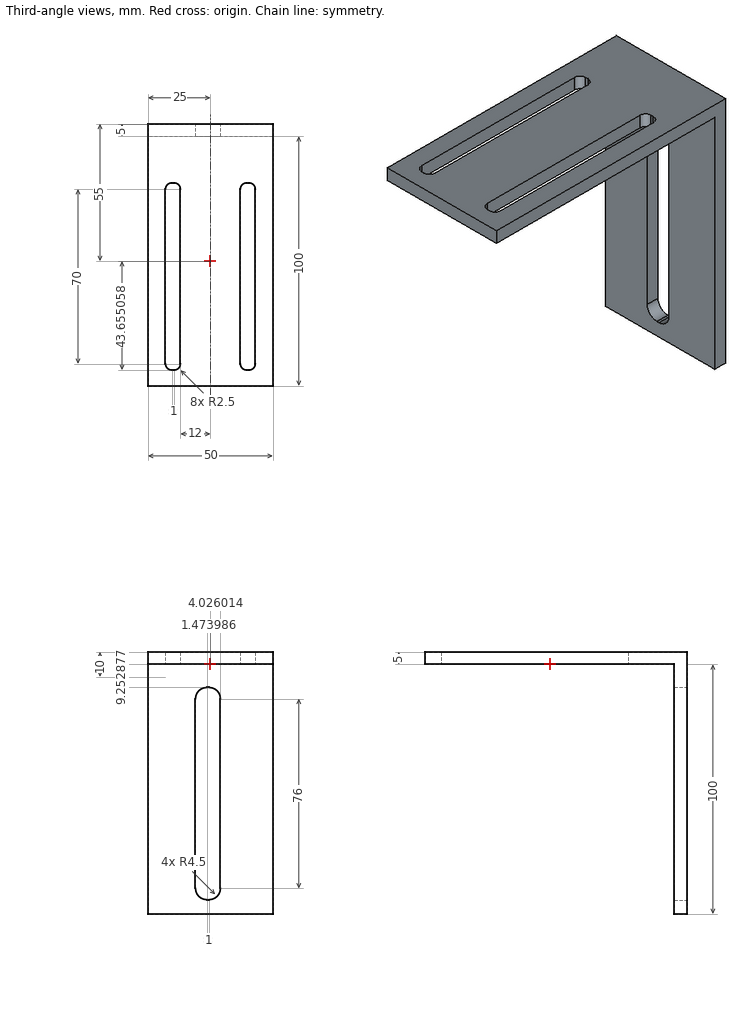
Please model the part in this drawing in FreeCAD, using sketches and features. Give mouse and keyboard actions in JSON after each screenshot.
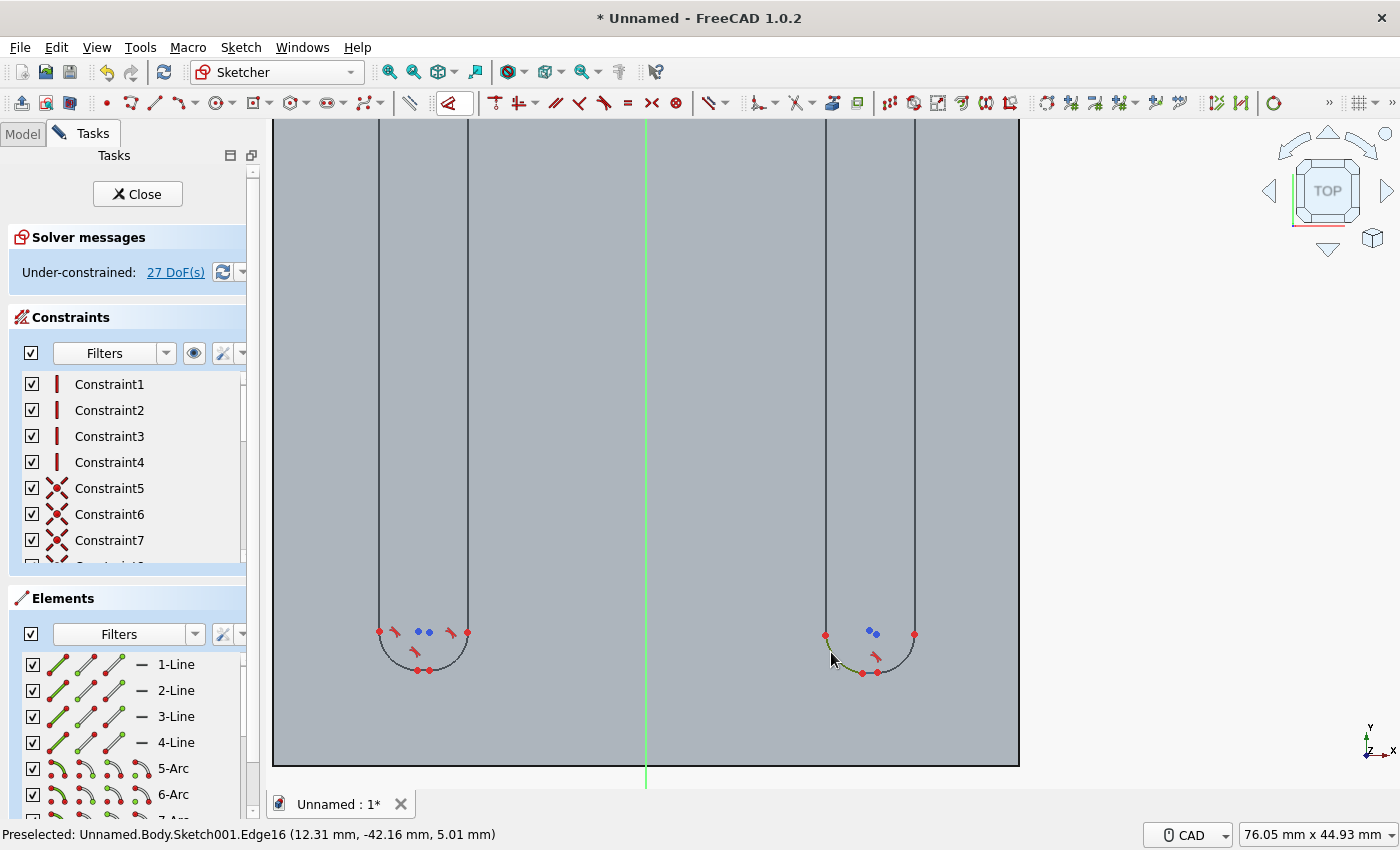
{"action": "left_click", "coordinate": [604, 104]}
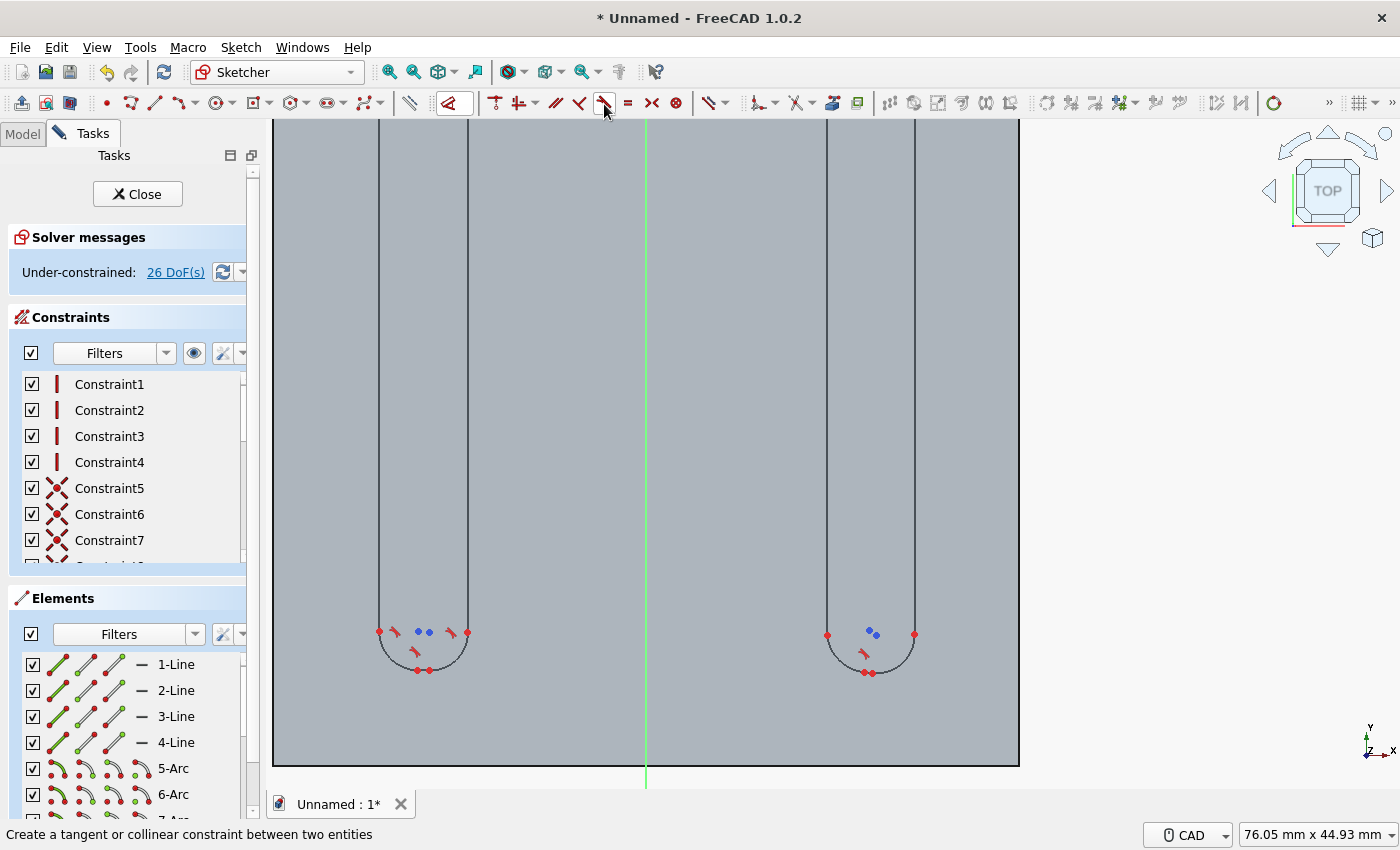
{"action": "left_click", "coordinate": [915, 322]}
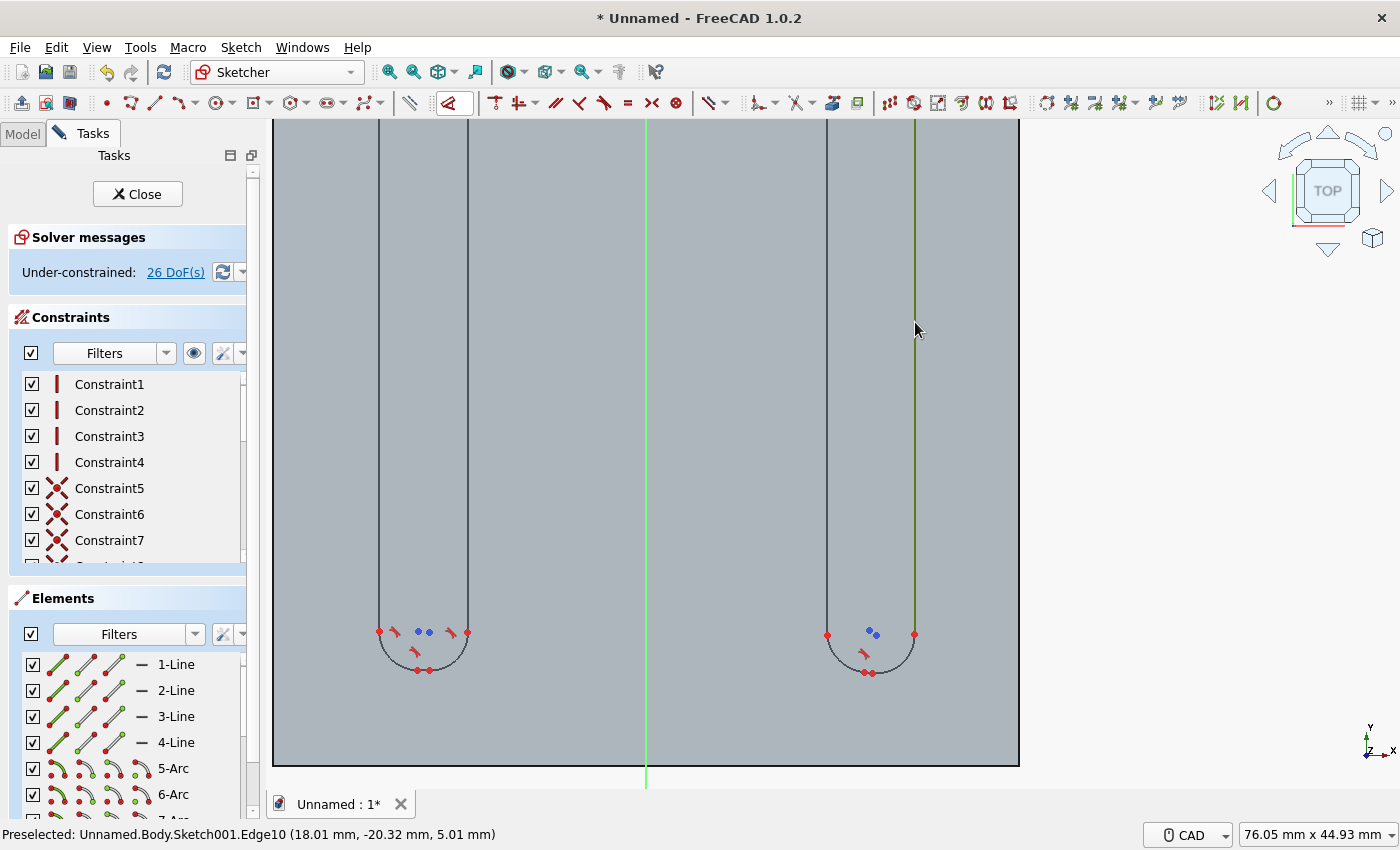
{"action": "left_click", "coordinate": [891, 670]}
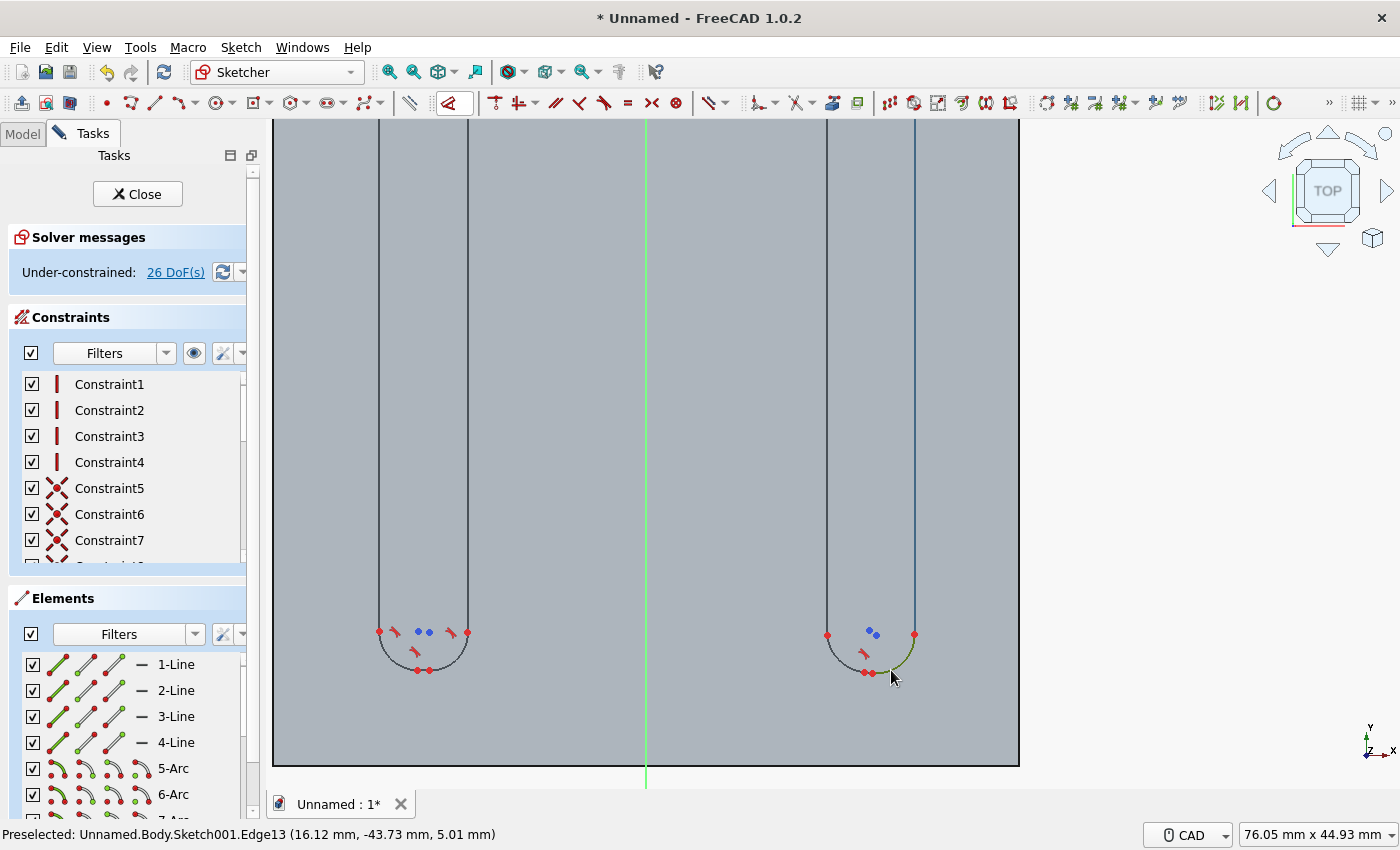
{"action": "key", "text": "t"}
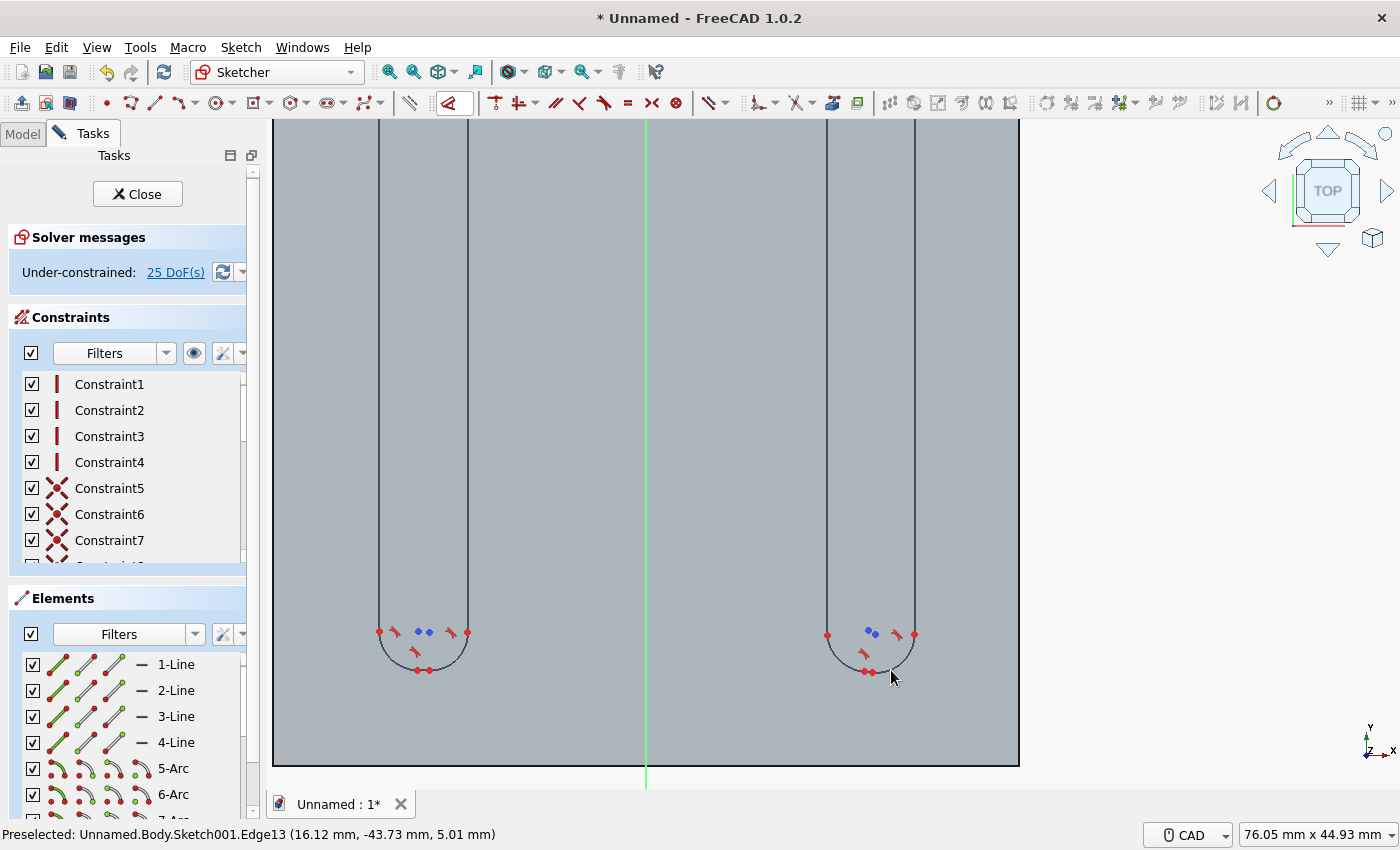
{"action": "left_click", "coordinate": [915, 322]}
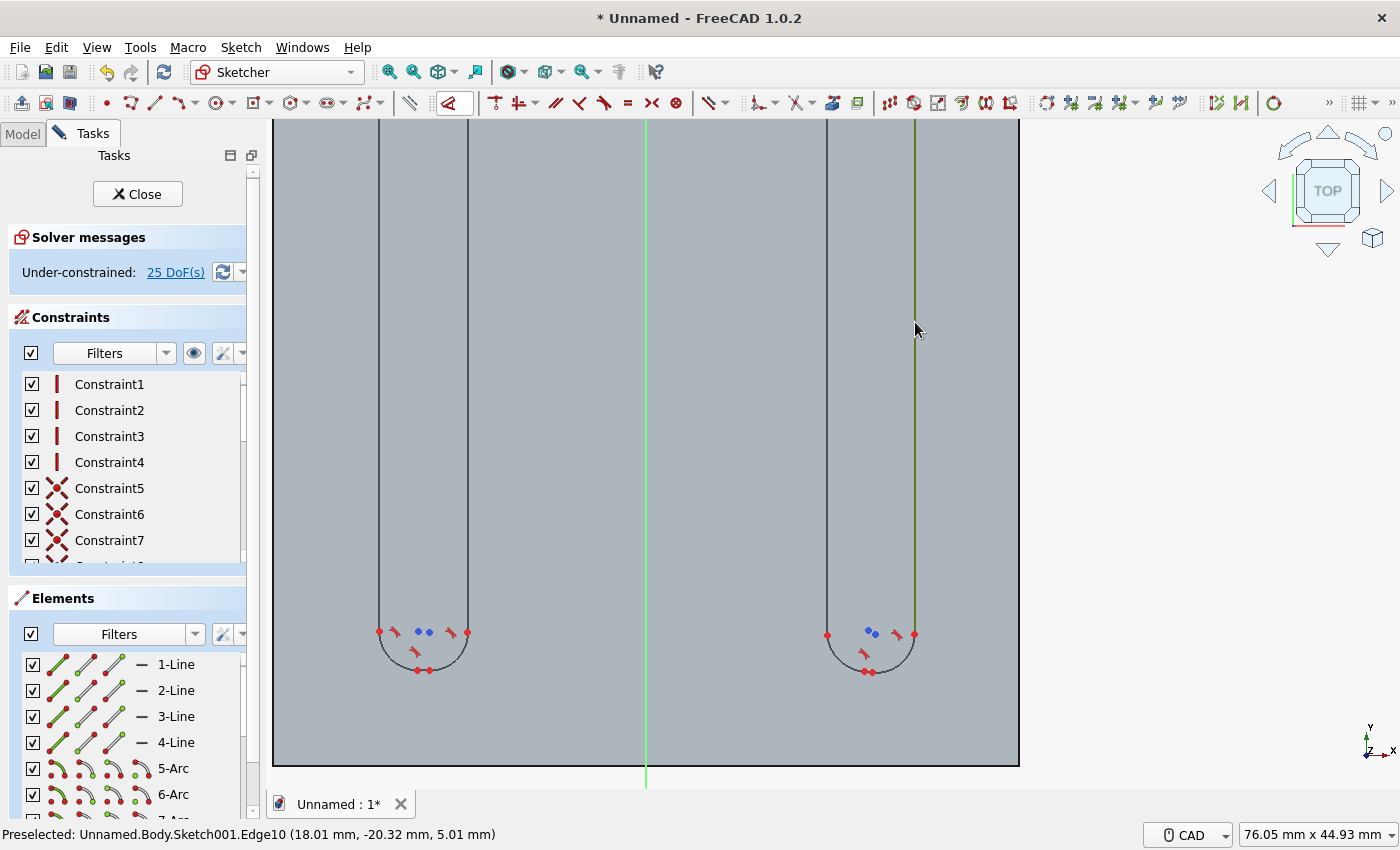
{"action": "scroll", "coordinate": [833, 653], "scroll_direction": "down", "scroll_amount": 5}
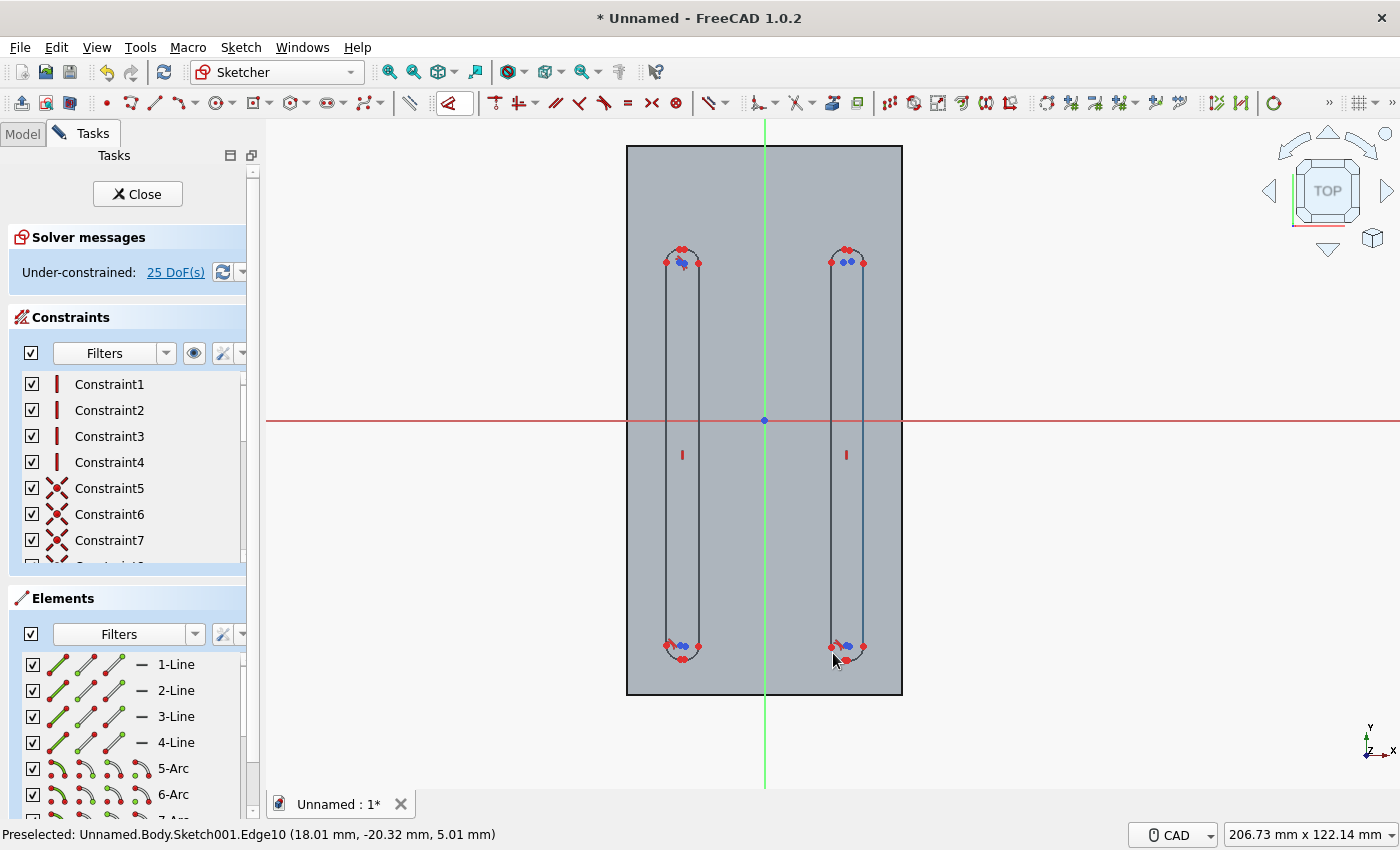
{"action": "scroll", "coordinate": [862, 257], "scroll_direction": "up", "scroll_amount": 4}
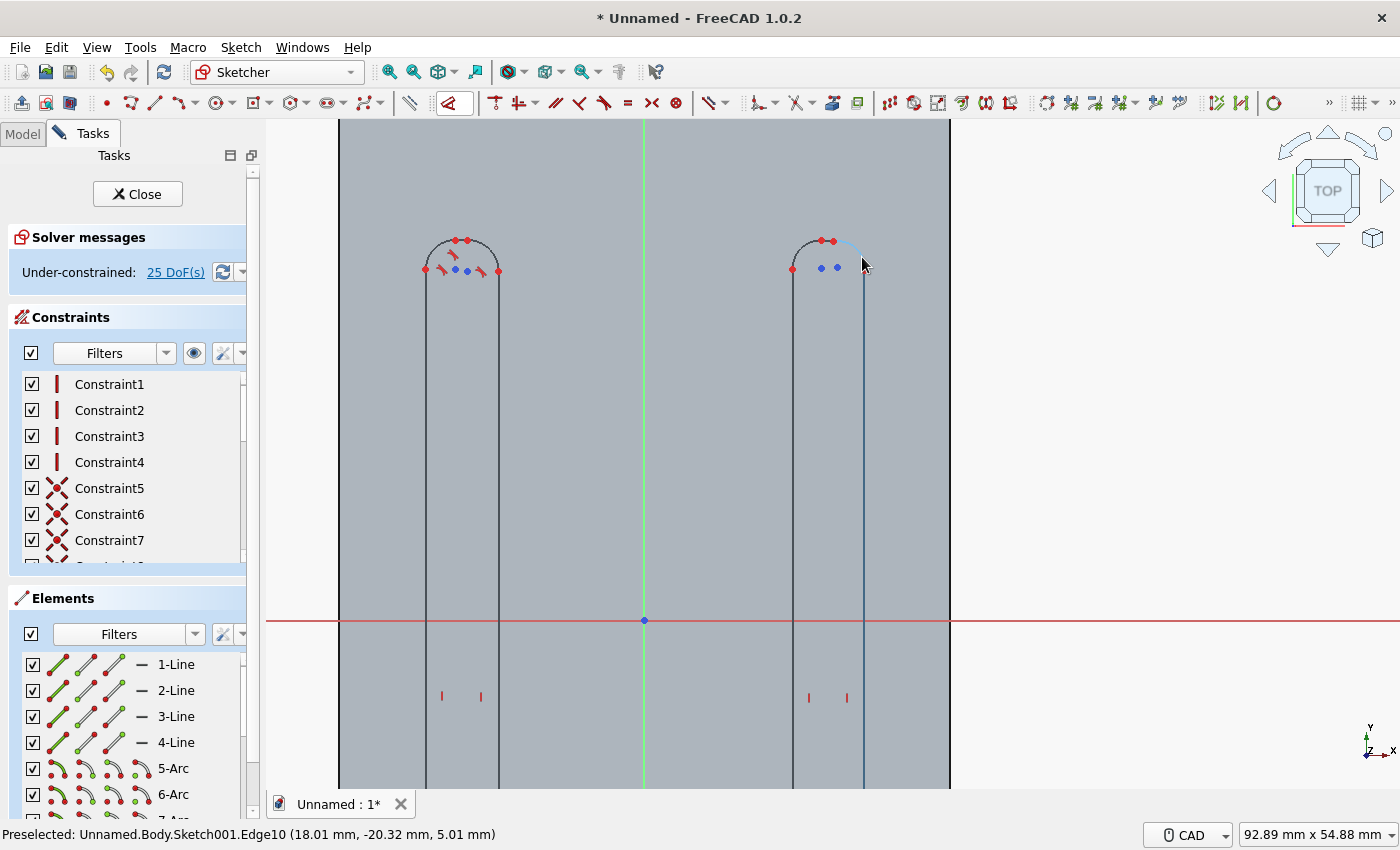
{"action": "left_click", "coordinate": [862, 256]}